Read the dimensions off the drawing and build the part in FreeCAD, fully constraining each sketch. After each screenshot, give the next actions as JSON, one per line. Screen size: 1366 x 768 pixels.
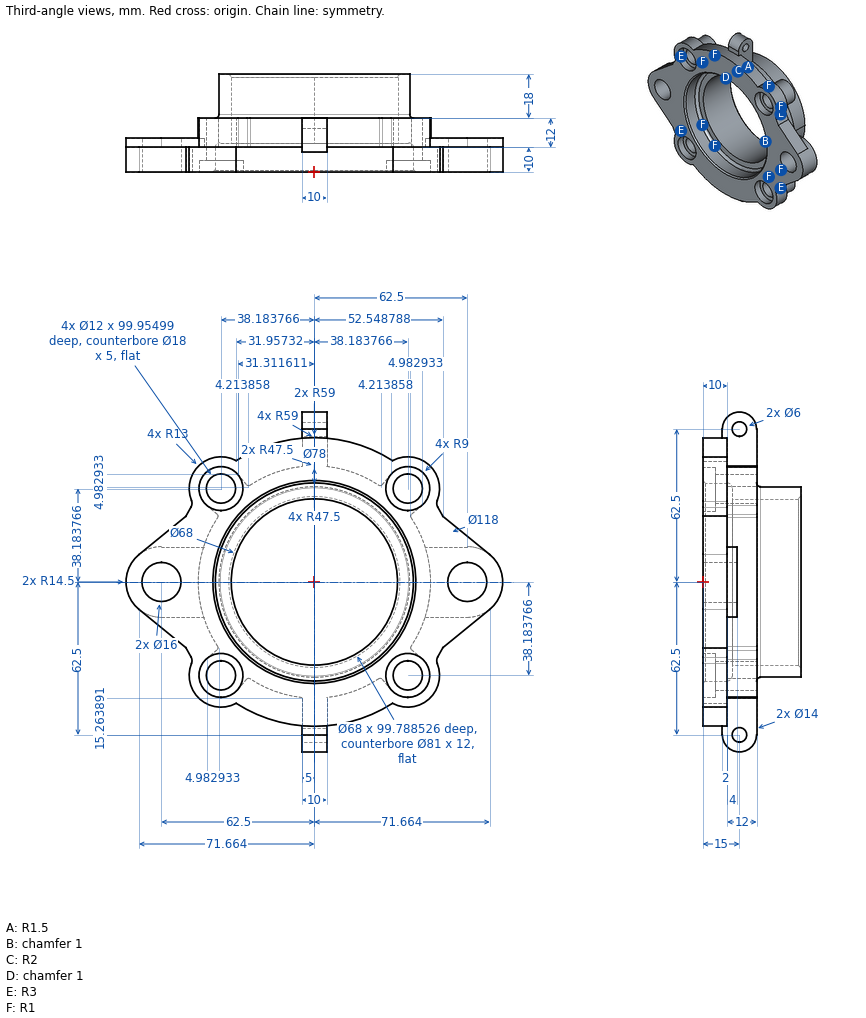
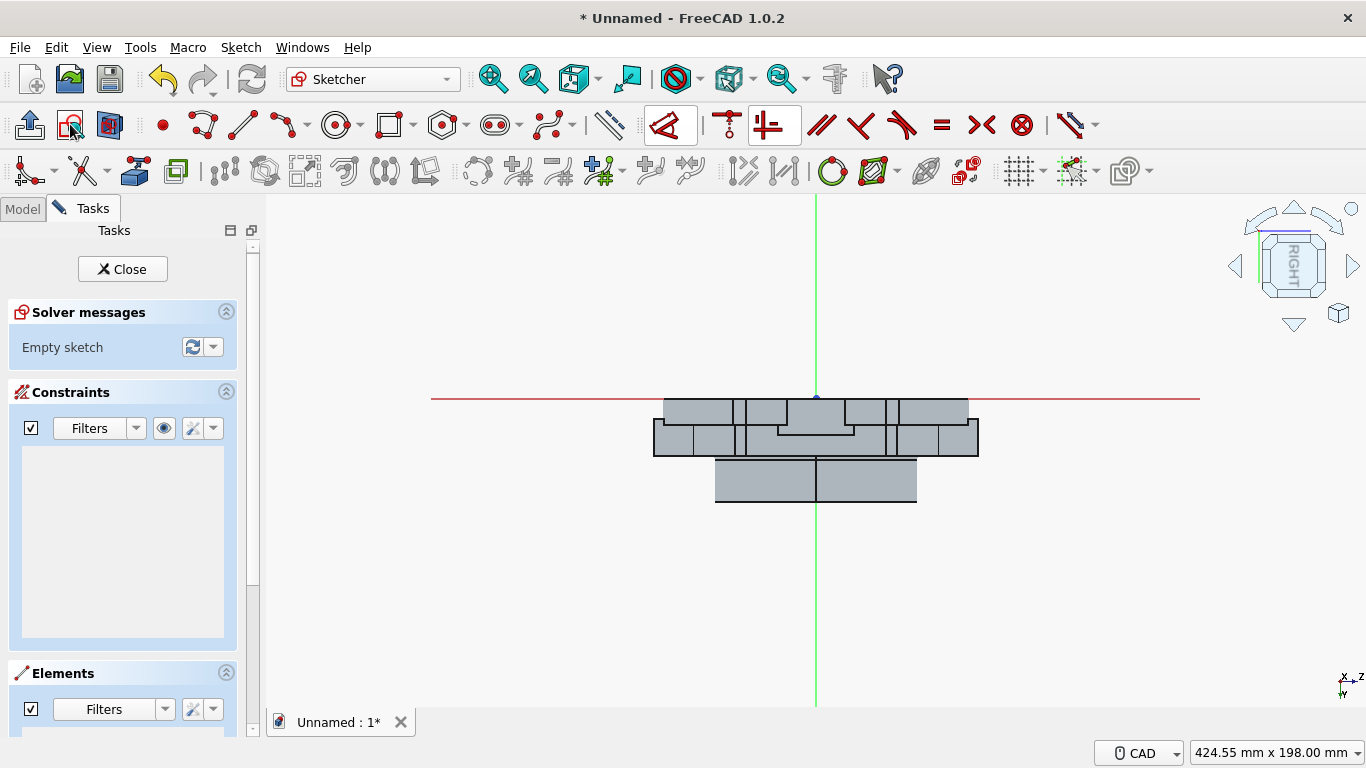
{"action": "left_click", "coordinate": [110, 126]}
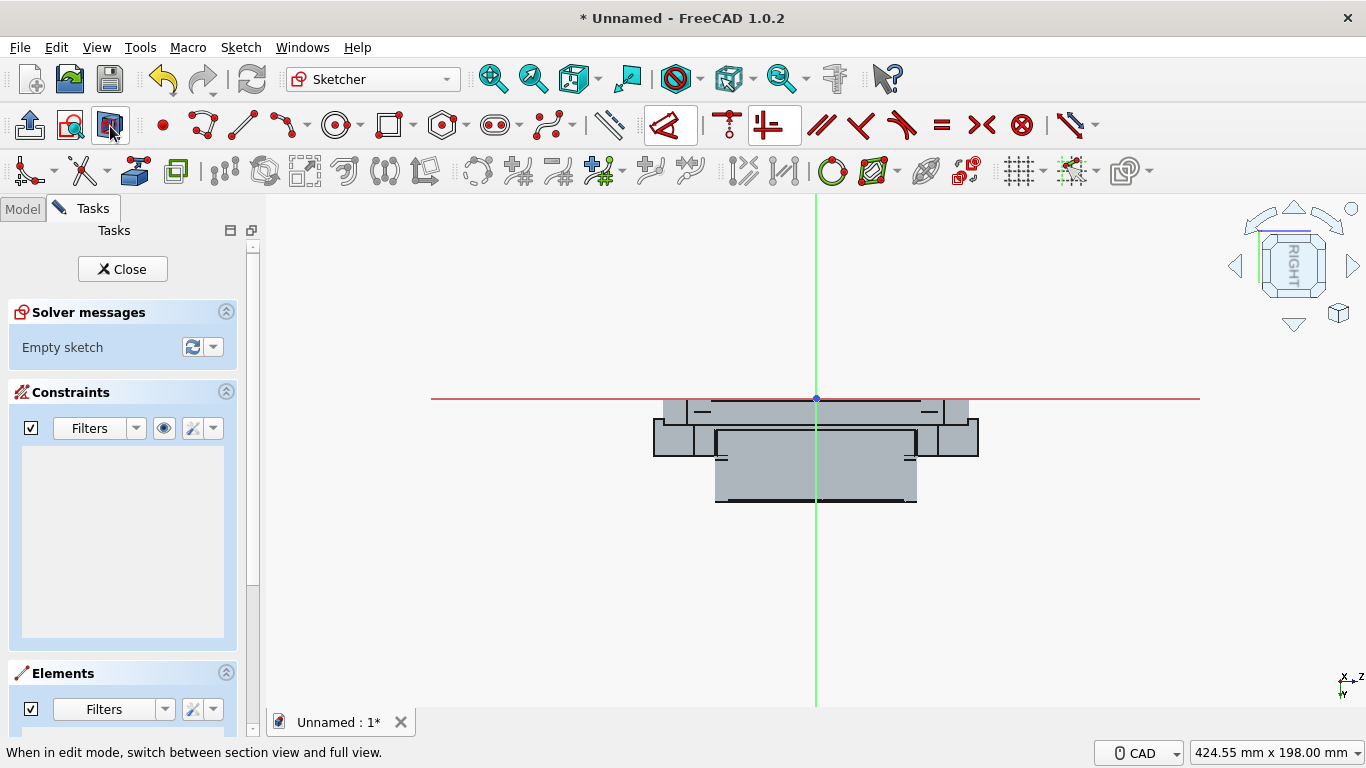
{"action": "scroll", "coordinate": [899, 399], "scroll_direction": "up", "scroll_amount": 3}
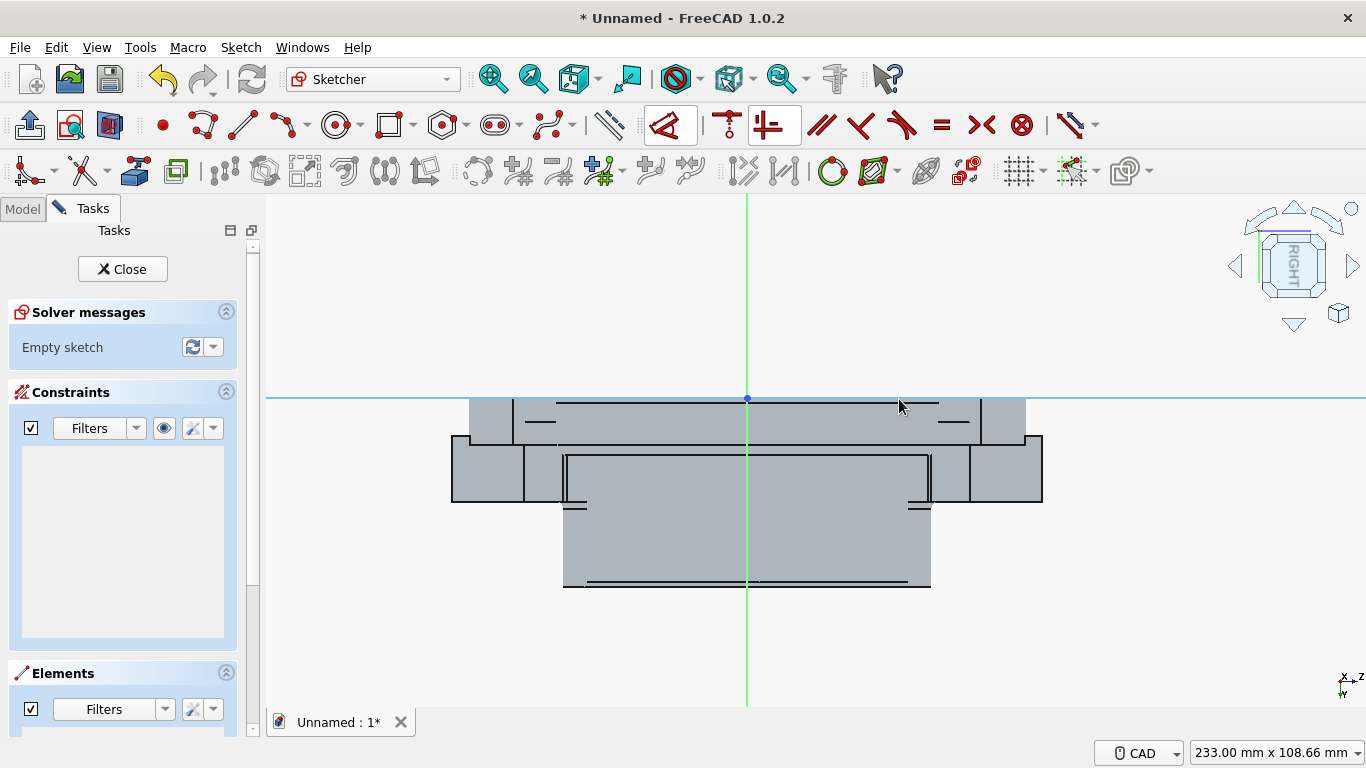
{"action": "left_click", "coordinate": [336, 126]}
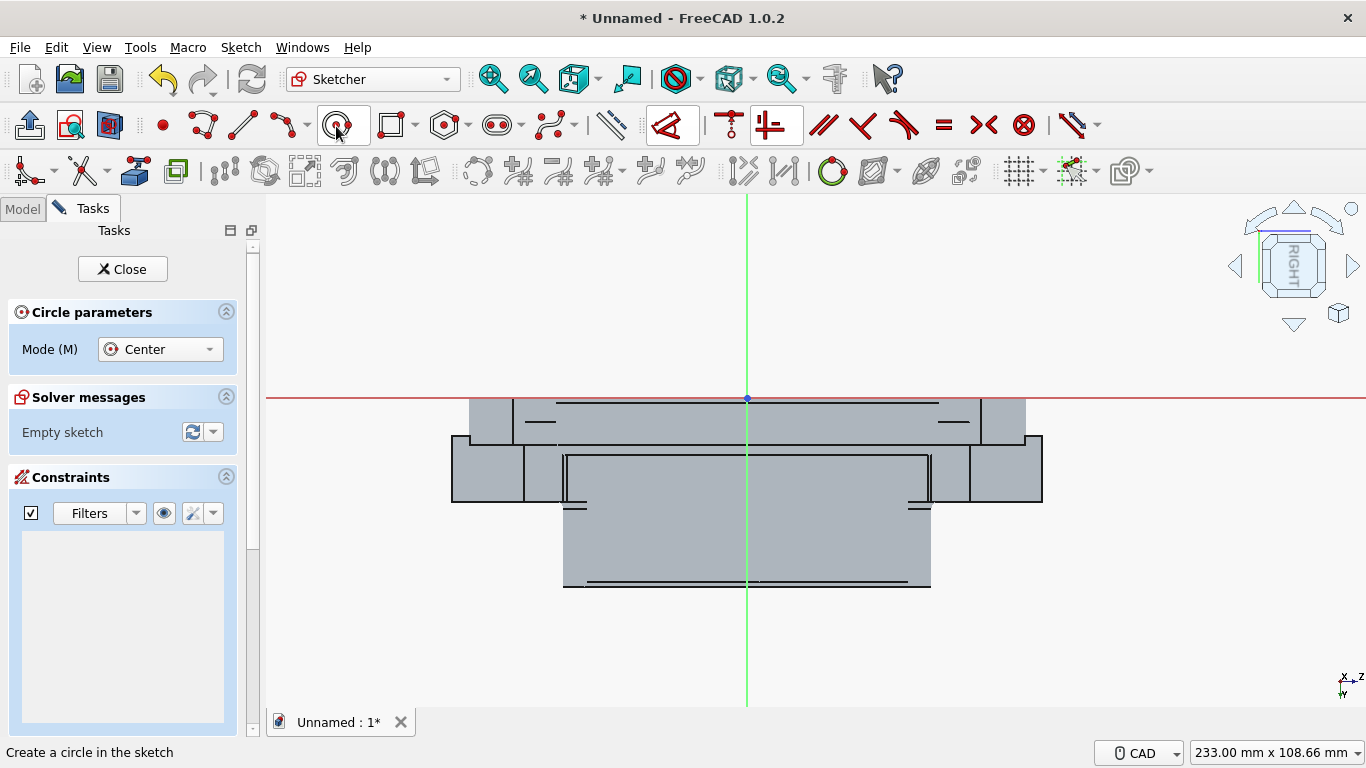
{"action": "left_click", "coordinate": [452, 469]}
{"action": "left_click", "coordinate": [476, 446]}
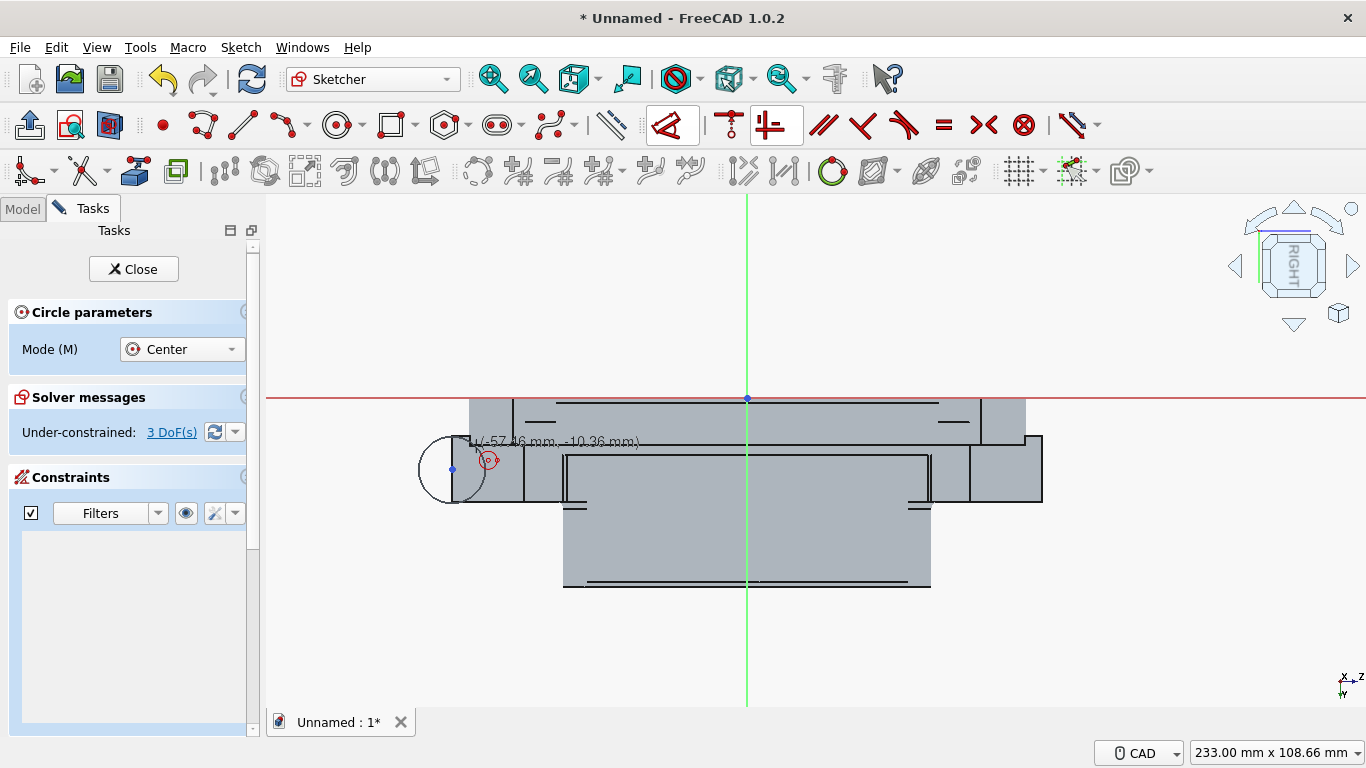
{"action": "left_click", "coordinate": [1042, 469]}
{"action": "left_click", "coordinate": [1066, 446]}
{"action": "key", "text": "Escape"}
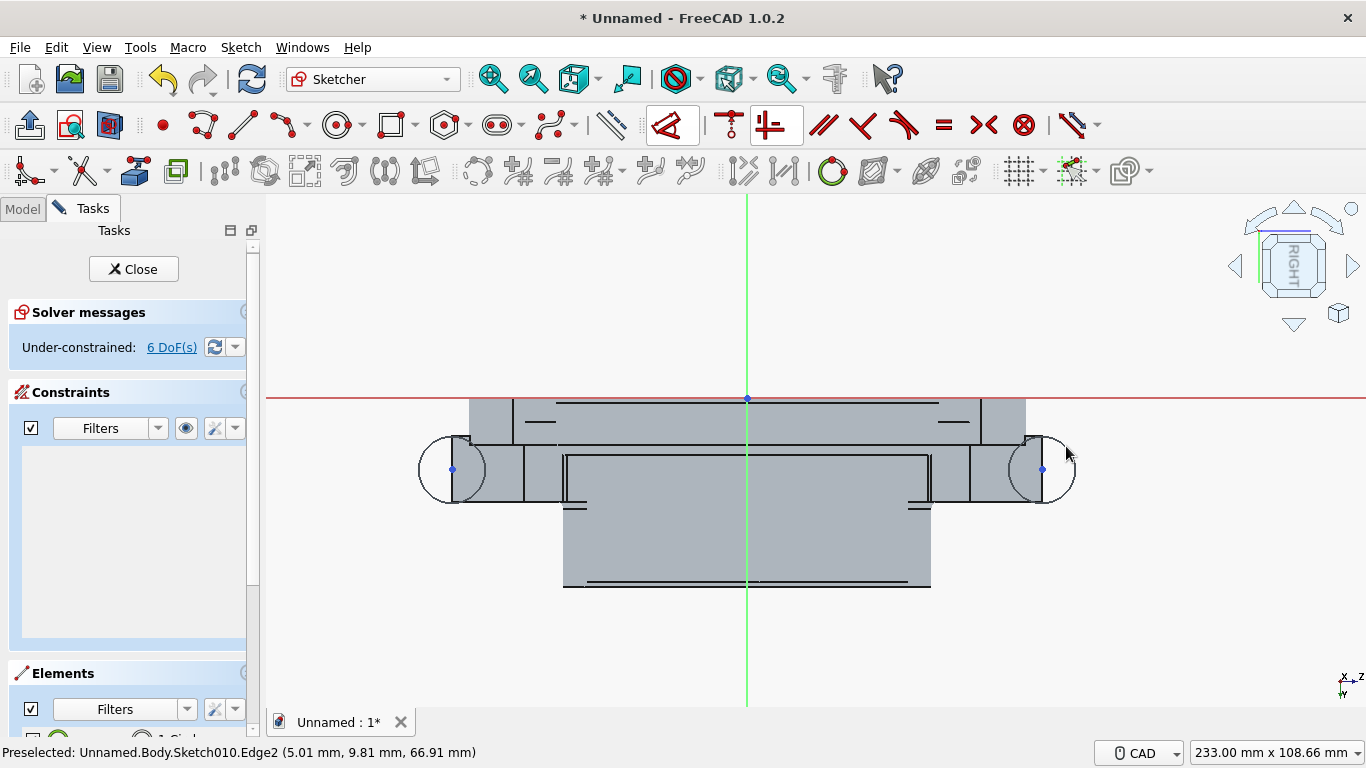
{"action": "left_click", "coordinate": [475, 446]}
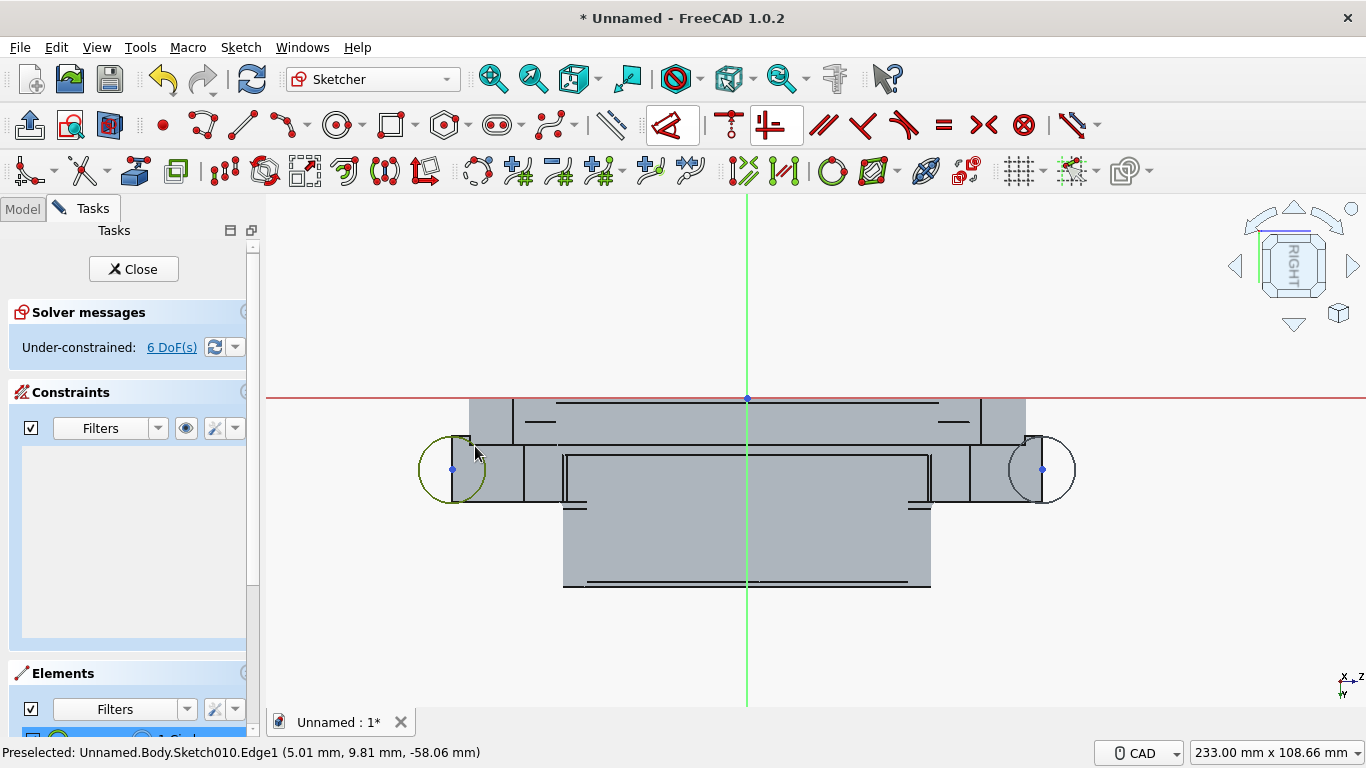
{"action": "left_click", "coordinate": [1065, 446]}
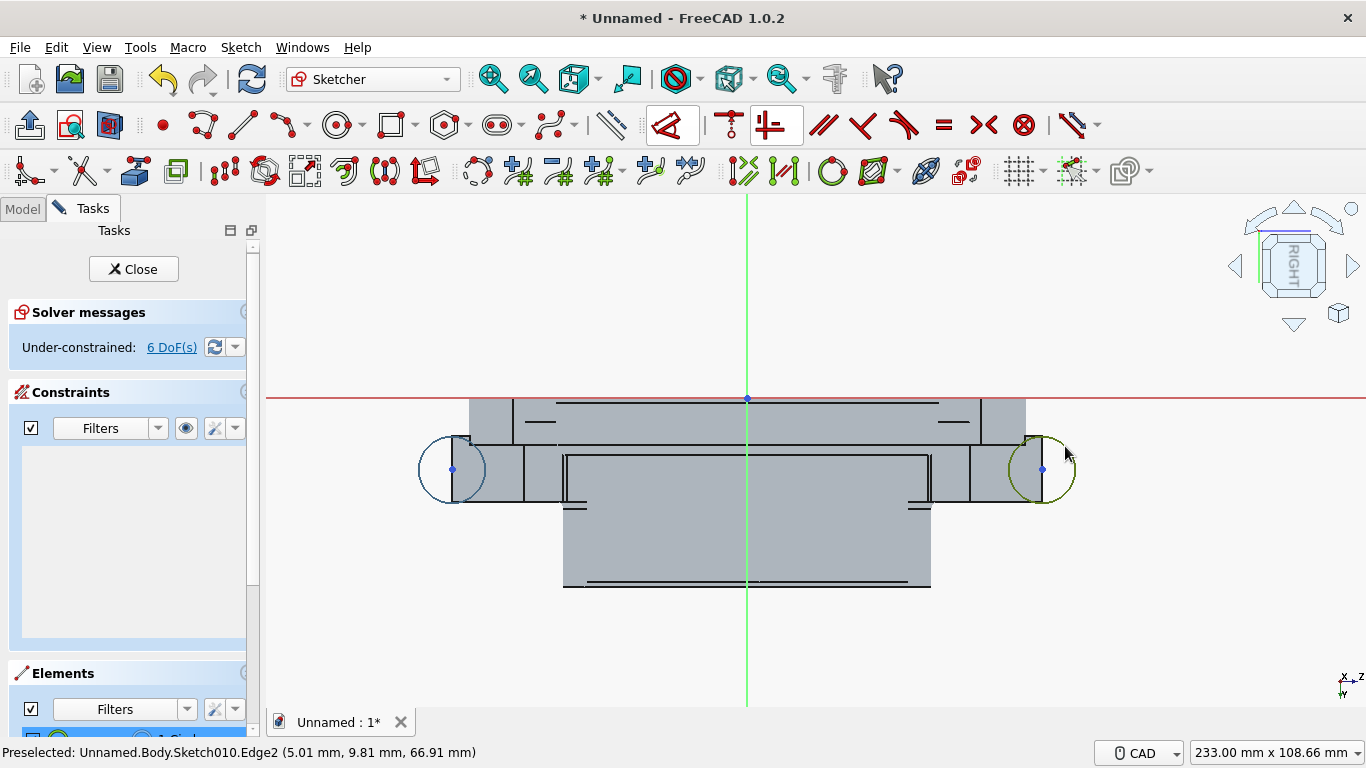
{"action": "left_click", "coordinate": [944, 126]}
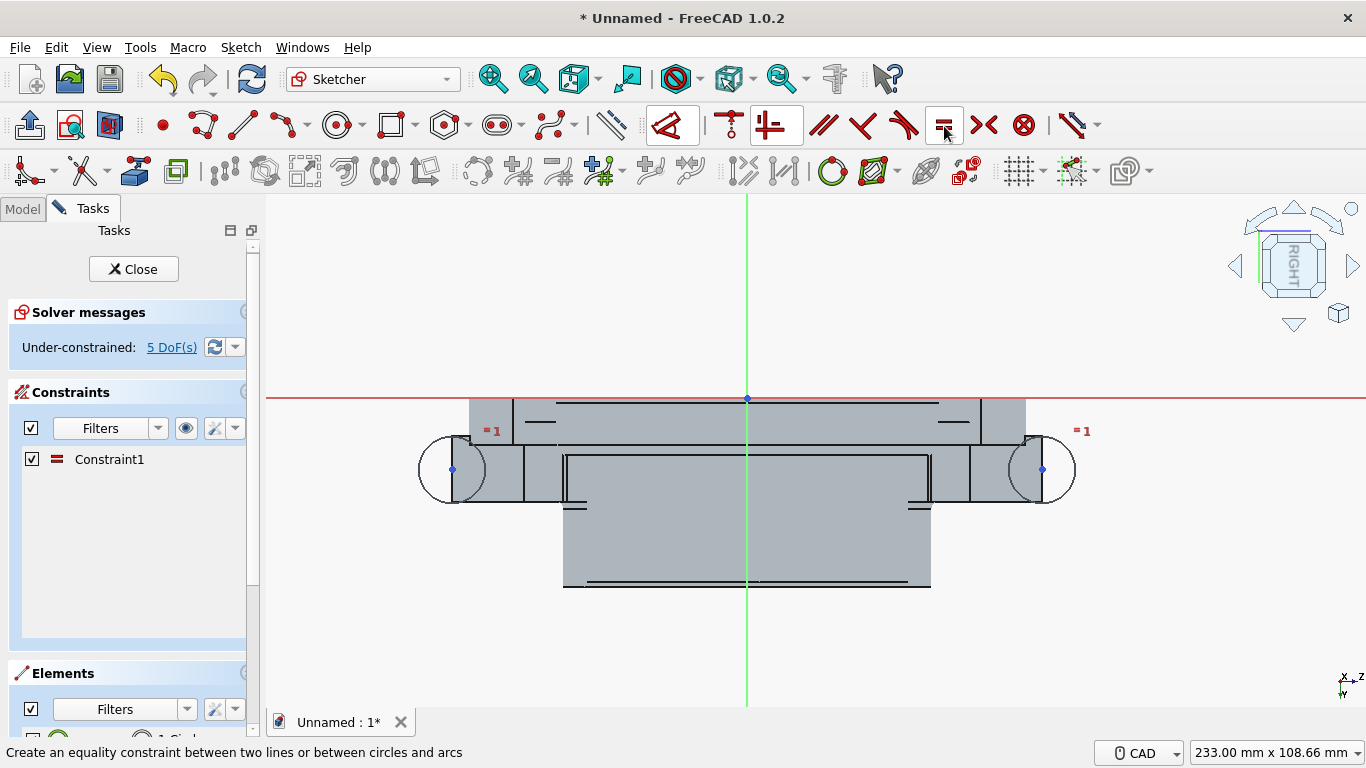
{"action": "left_click", "coordinate": [452, 470]}